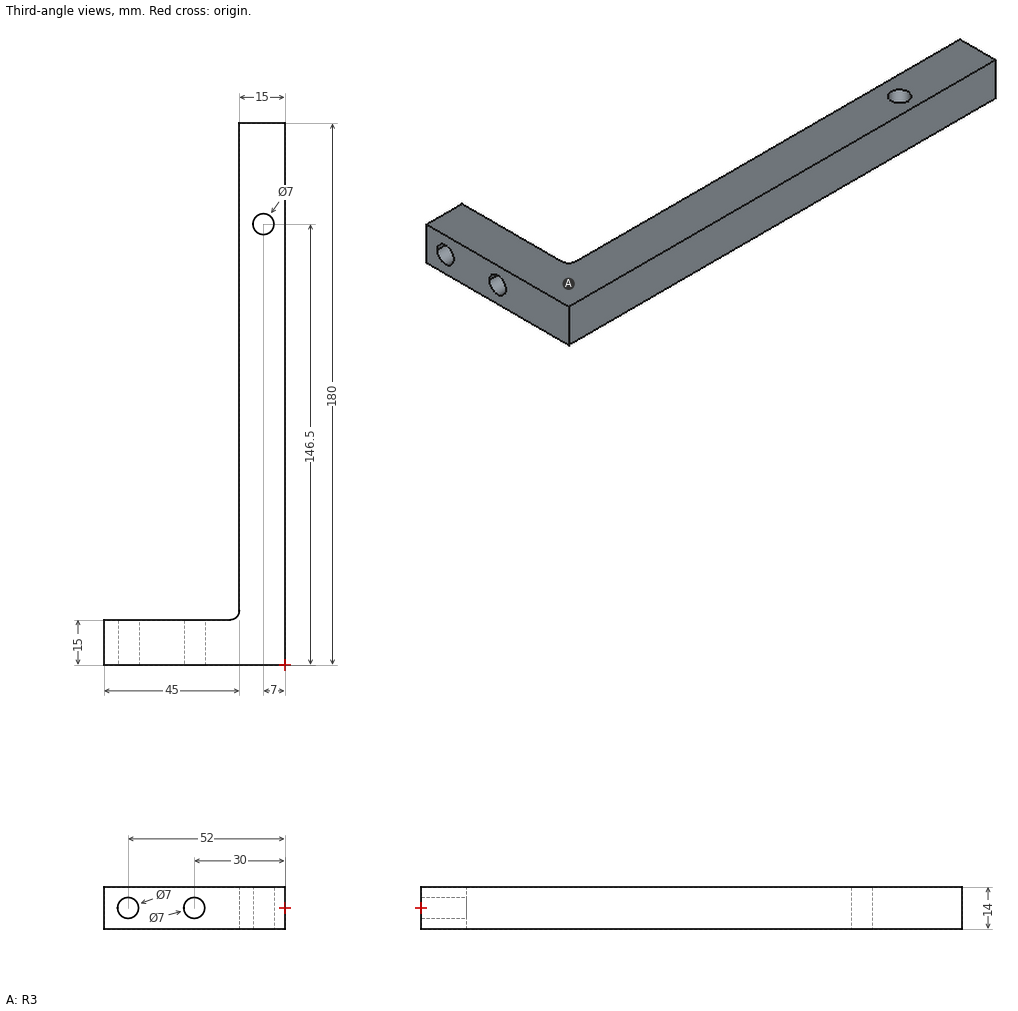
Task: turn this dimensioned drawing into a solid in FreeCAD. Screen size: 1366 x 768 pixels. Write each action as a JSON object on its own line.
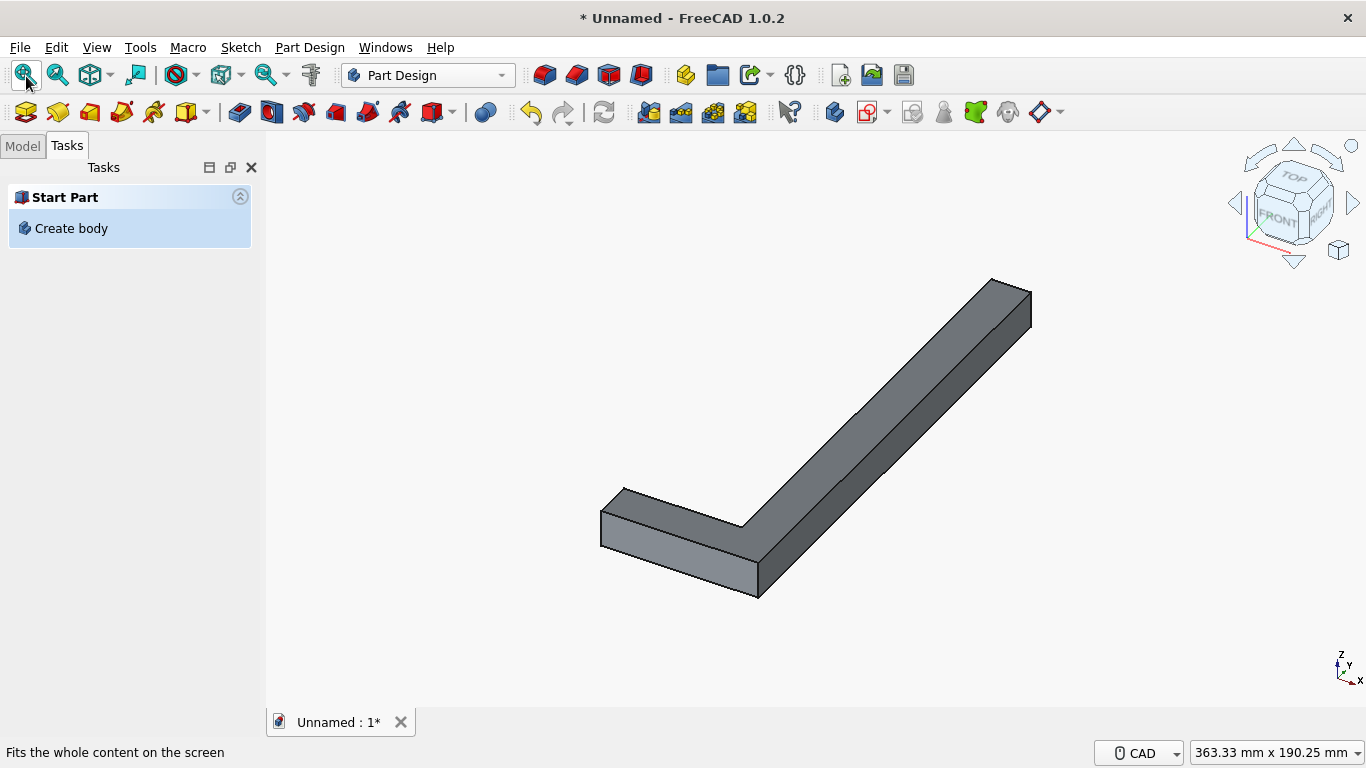
{"action": "key", "text": "0"}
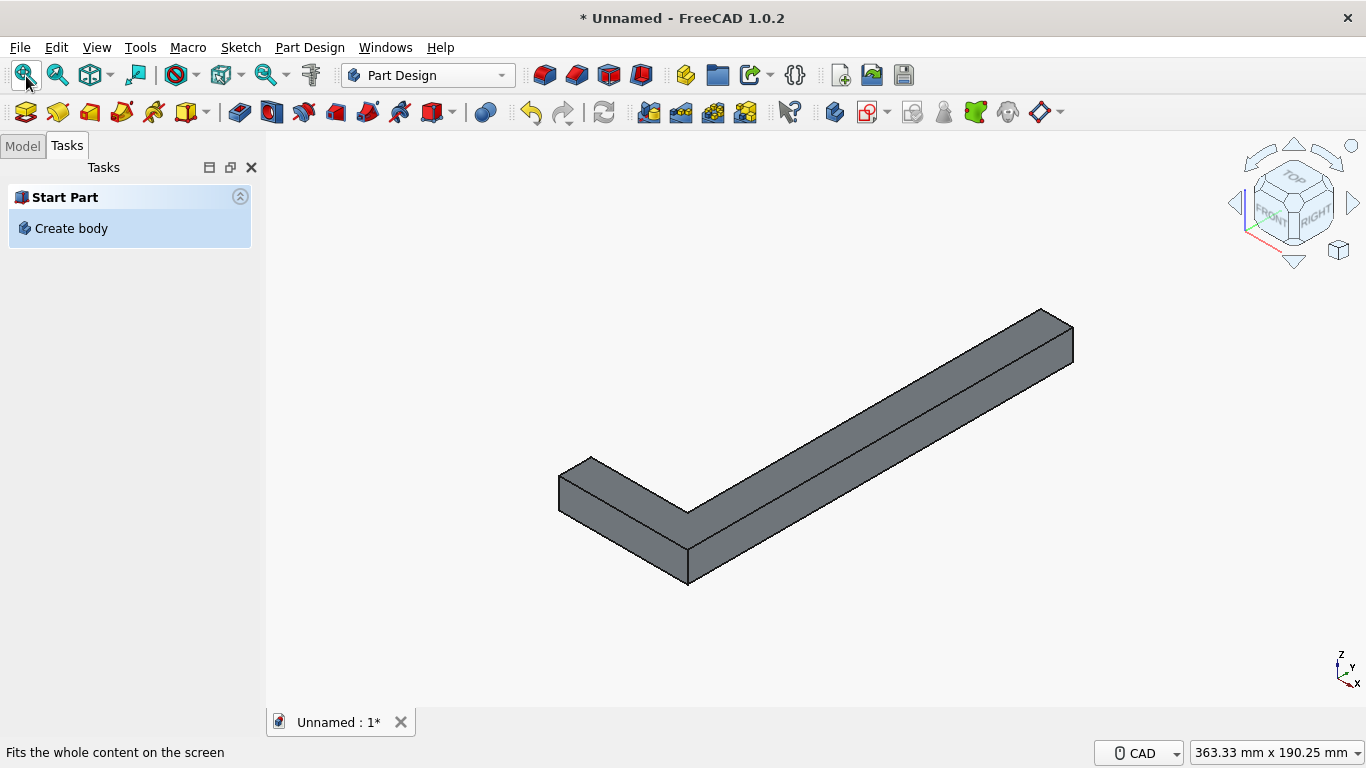
{"action": "key", "text": "2"}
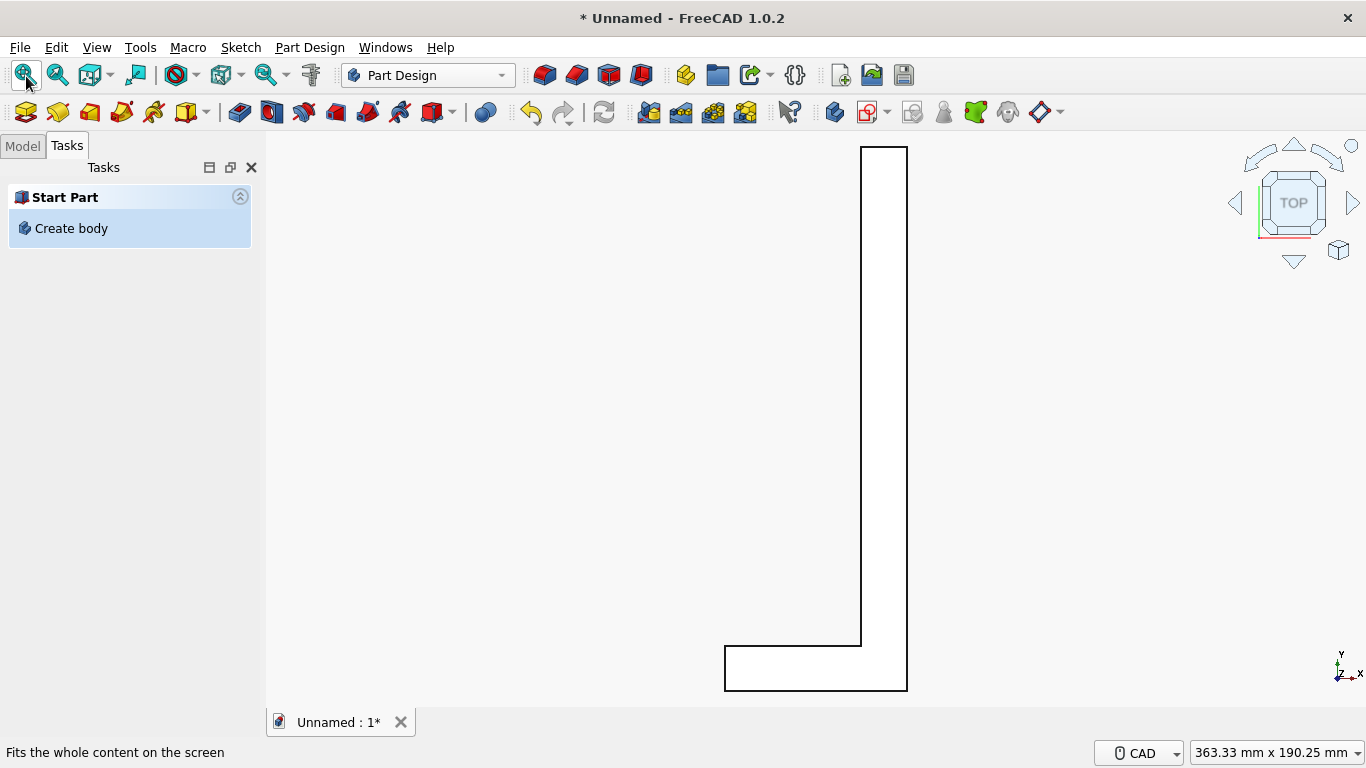
{"action": "key", "text": "1"}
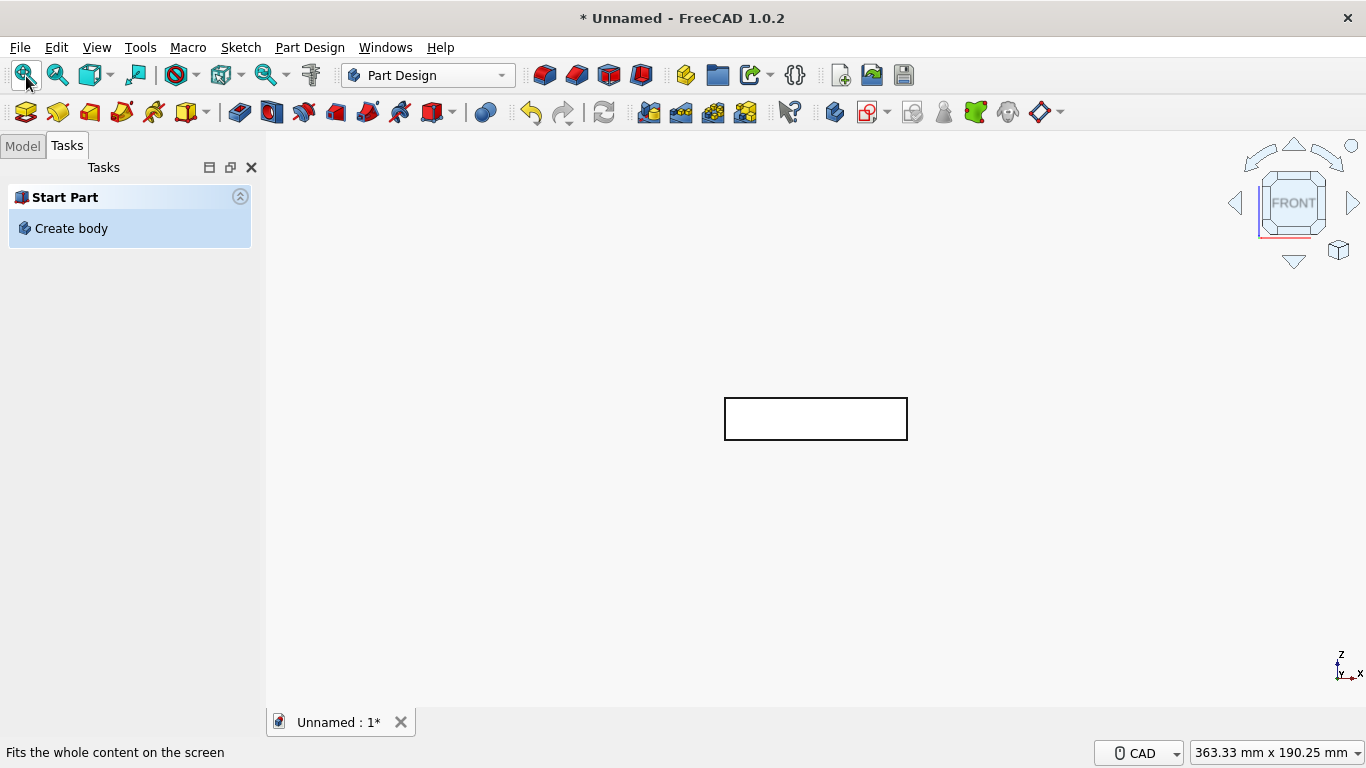
{"action": "left_click", "coordinate": [26, 76]}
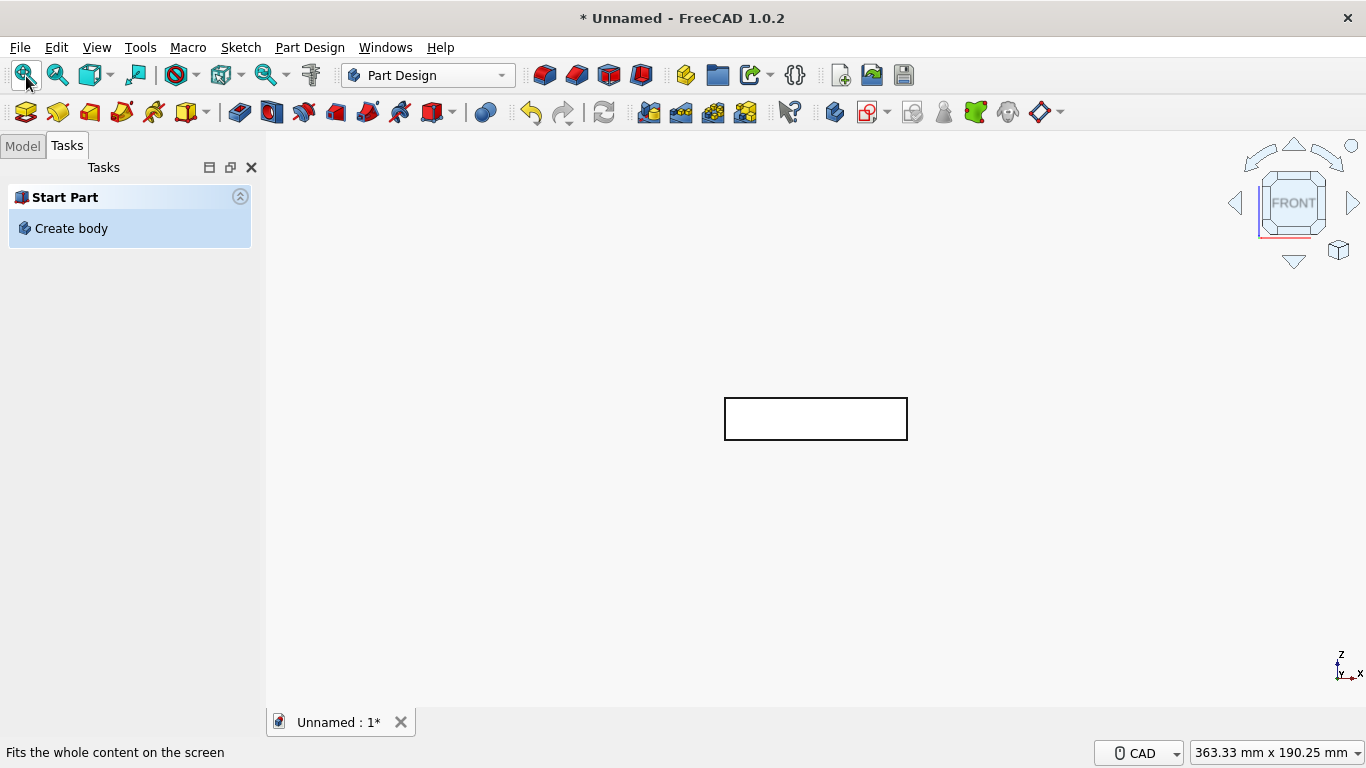
{"action": "key", "text": "3"}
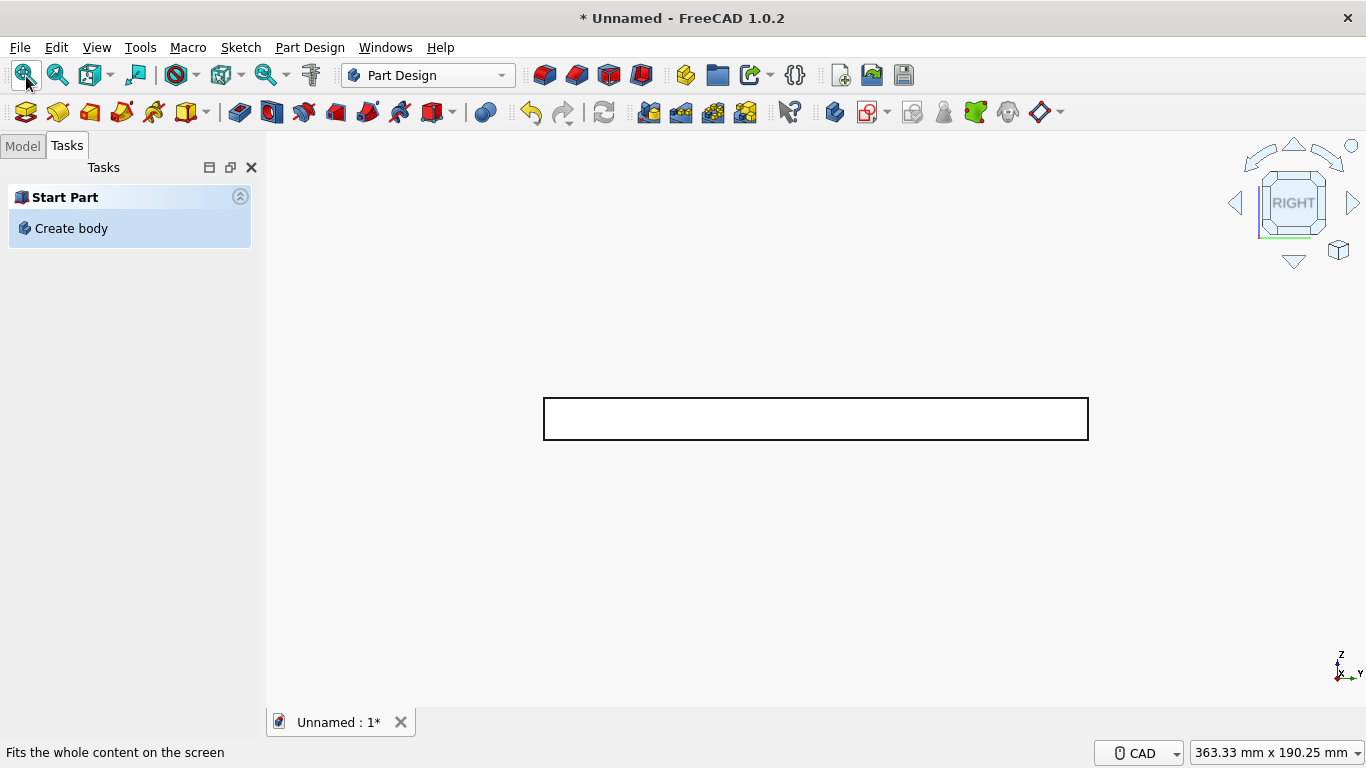
{"action": "key", "text": "5"}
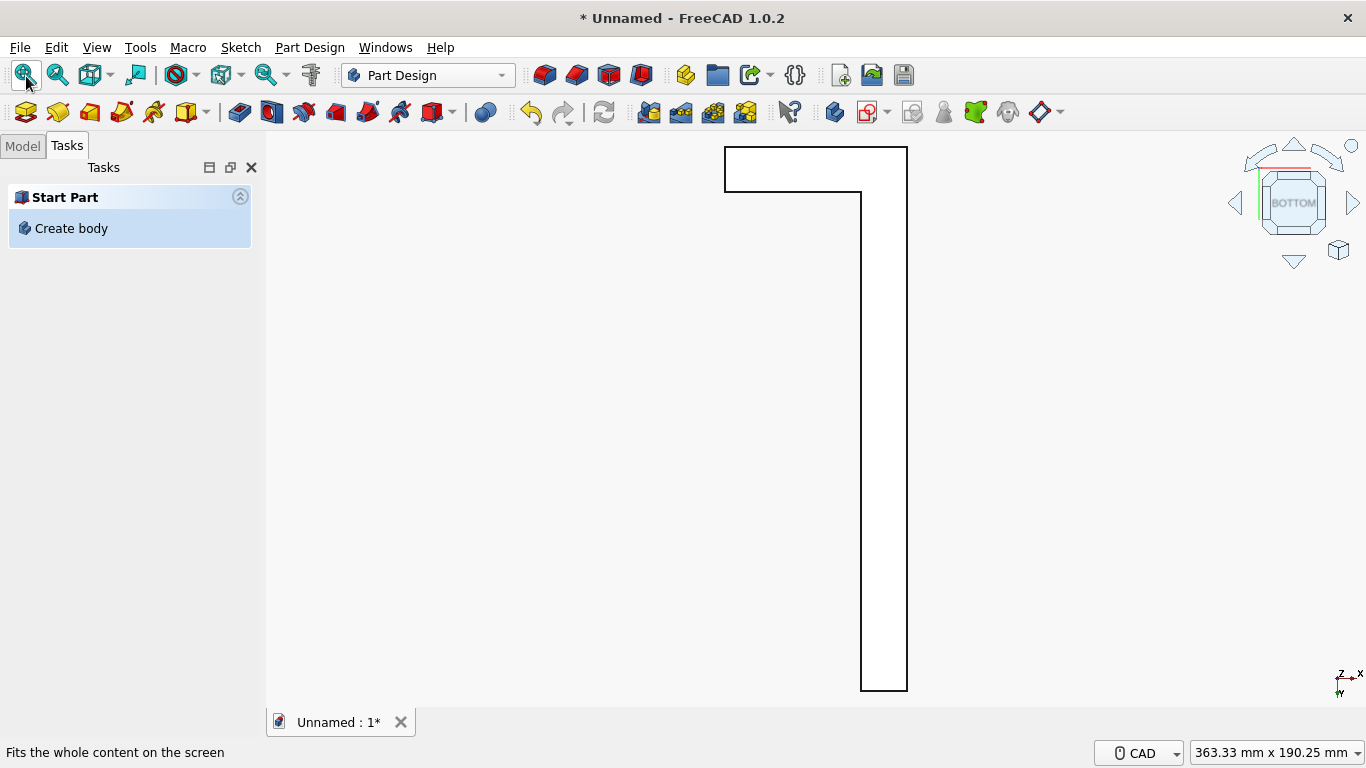
{"action": "key", "text": "4"}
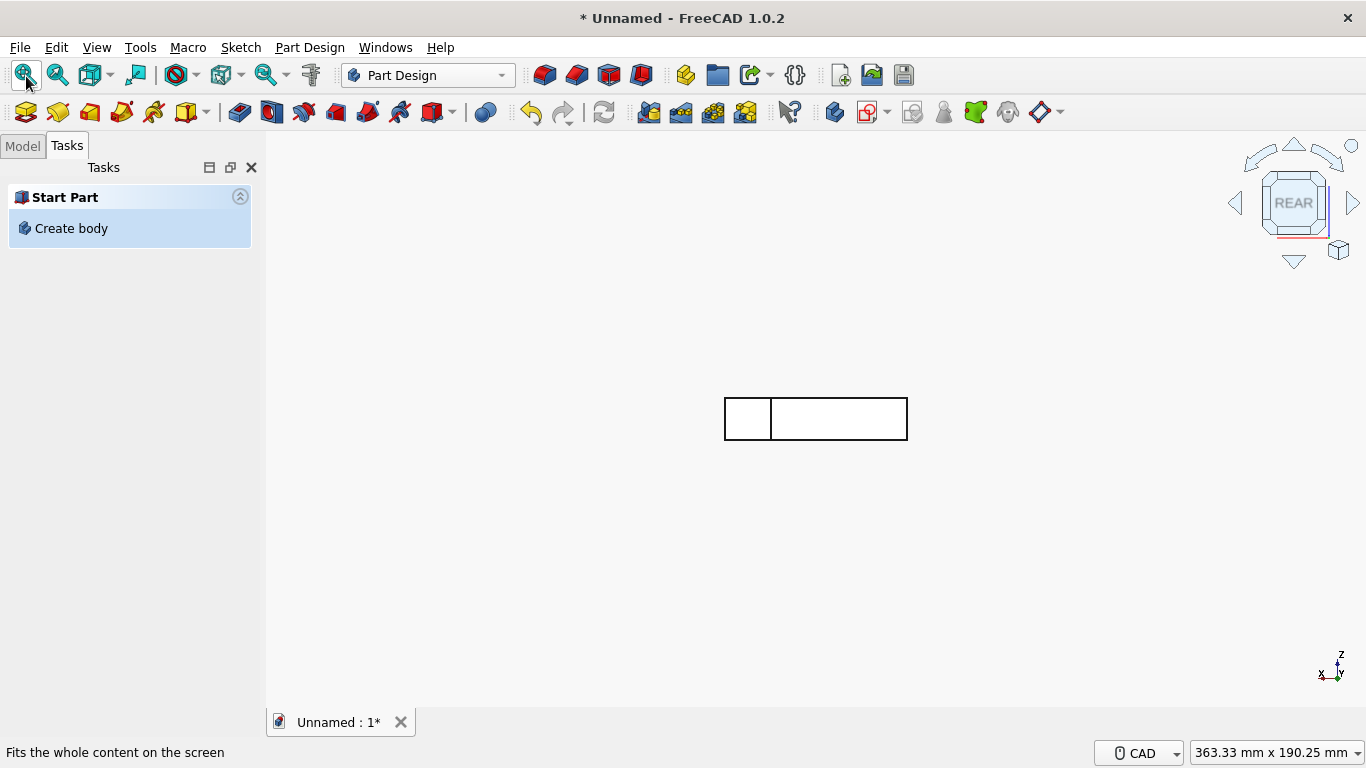
{"action": "left_click", "coordinate": [26, 76]}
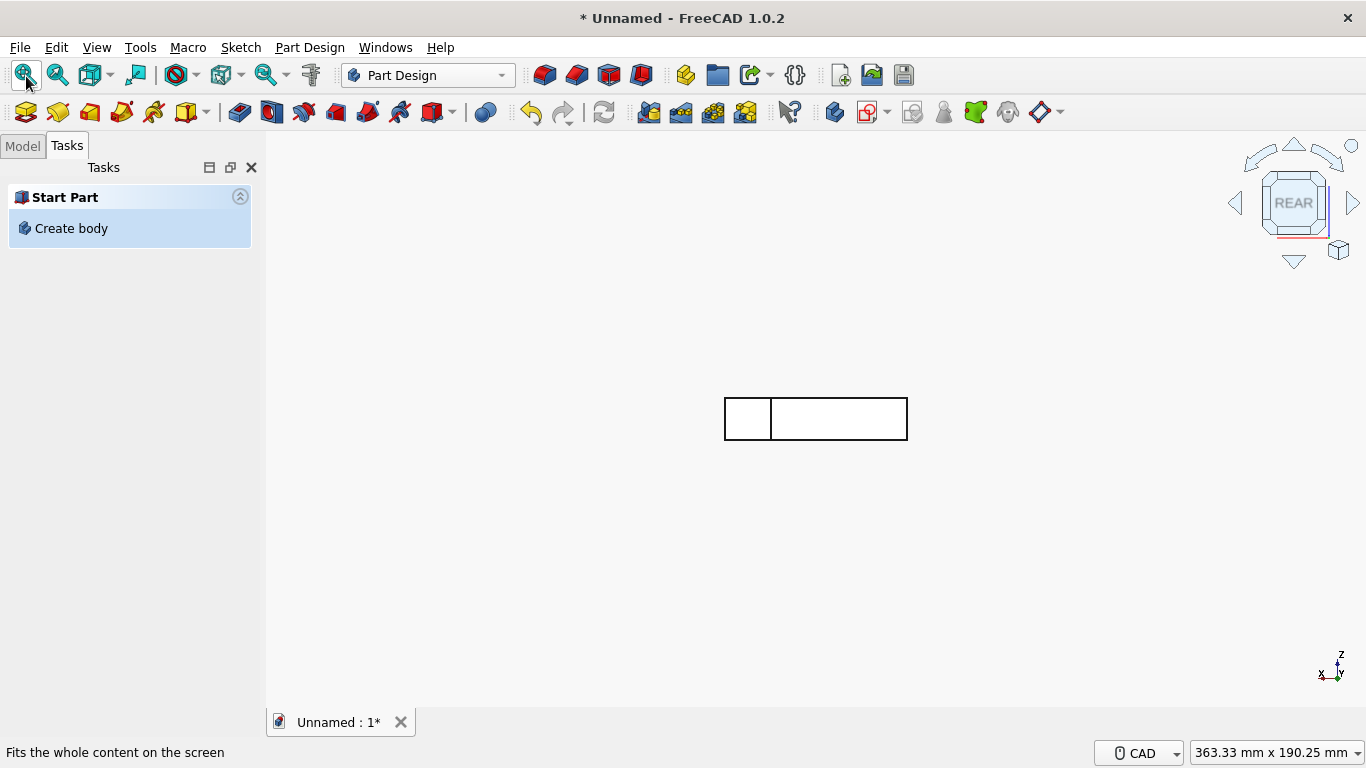
{"action": "key", "text": "6"}